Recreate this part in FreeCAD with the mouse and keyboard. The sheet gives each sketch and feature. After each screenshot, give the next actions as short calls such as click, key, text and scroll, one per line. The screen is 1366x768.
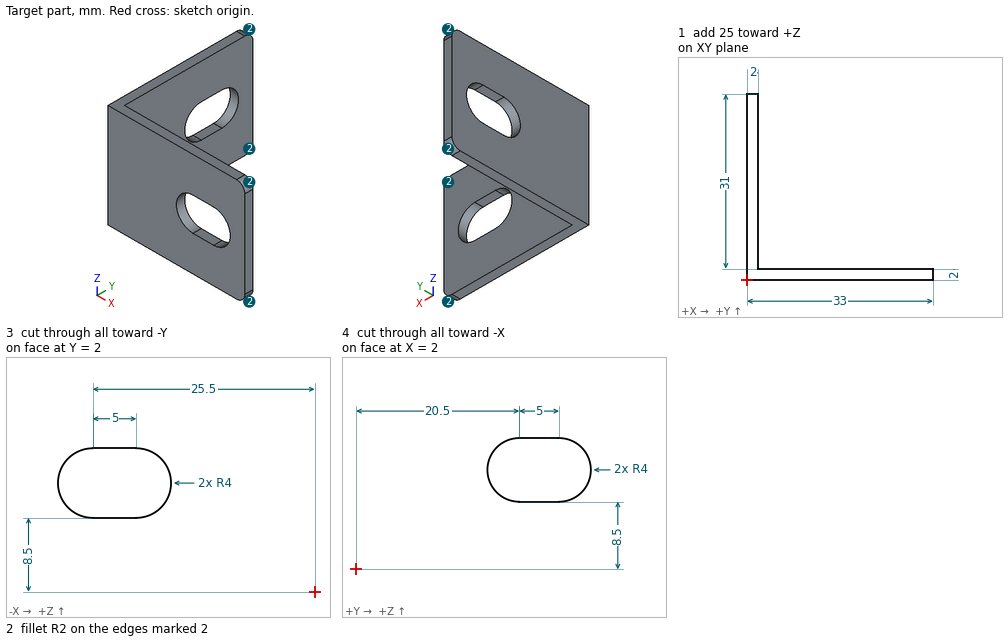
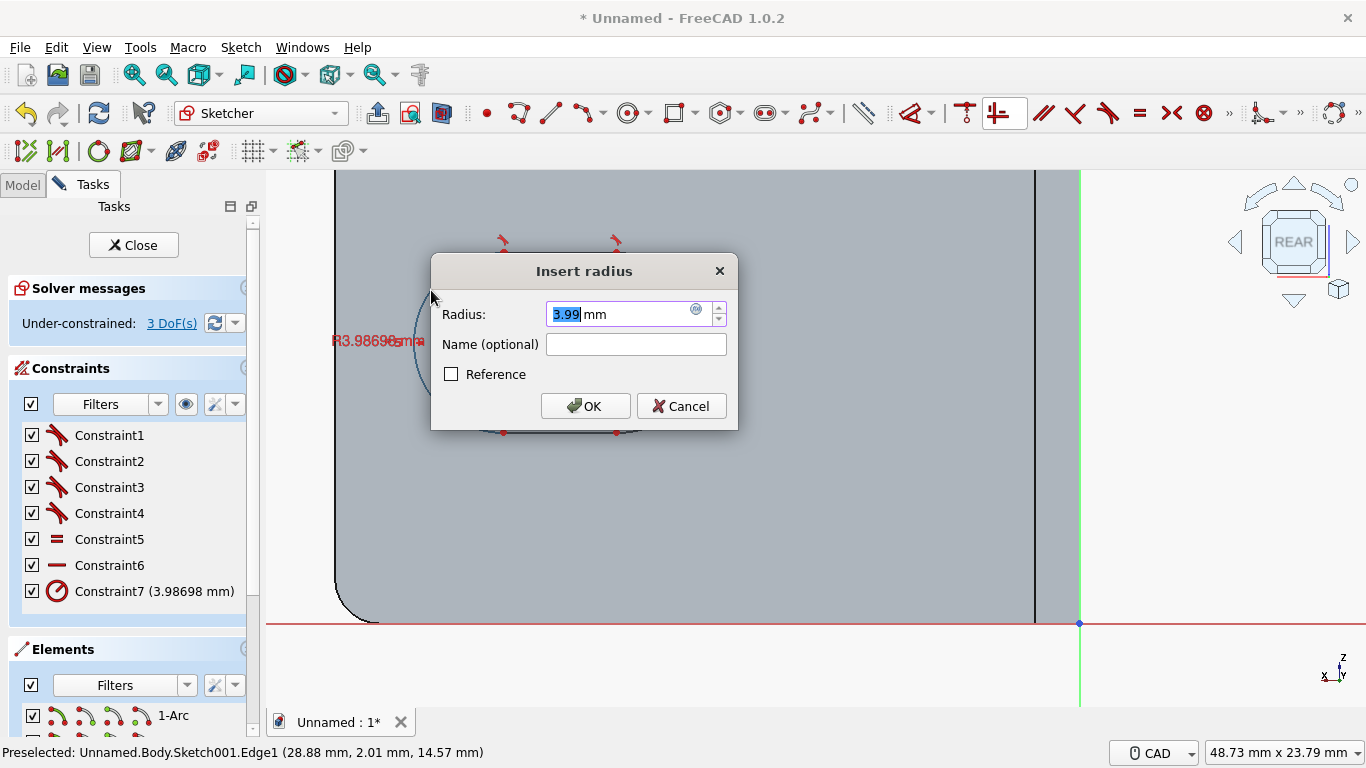
text(4)
key(Return)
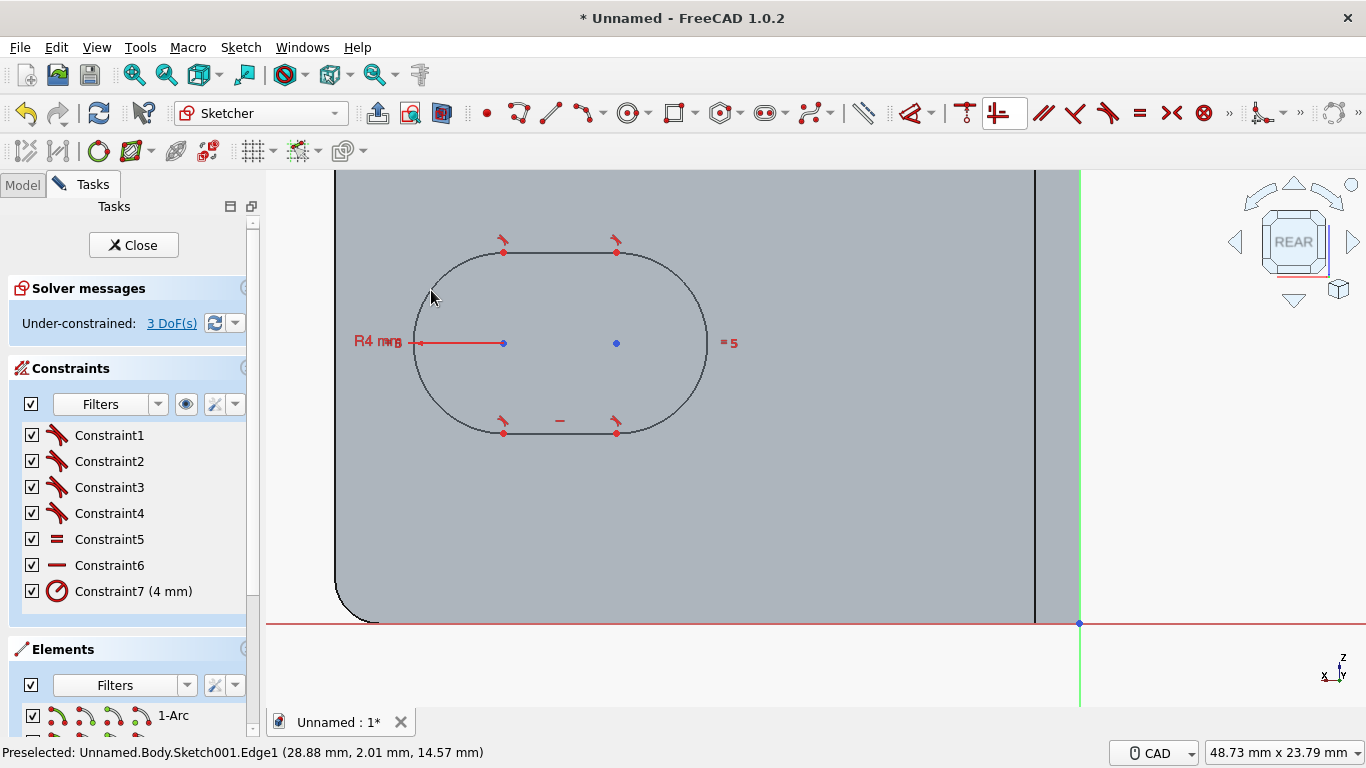
click(538, 253)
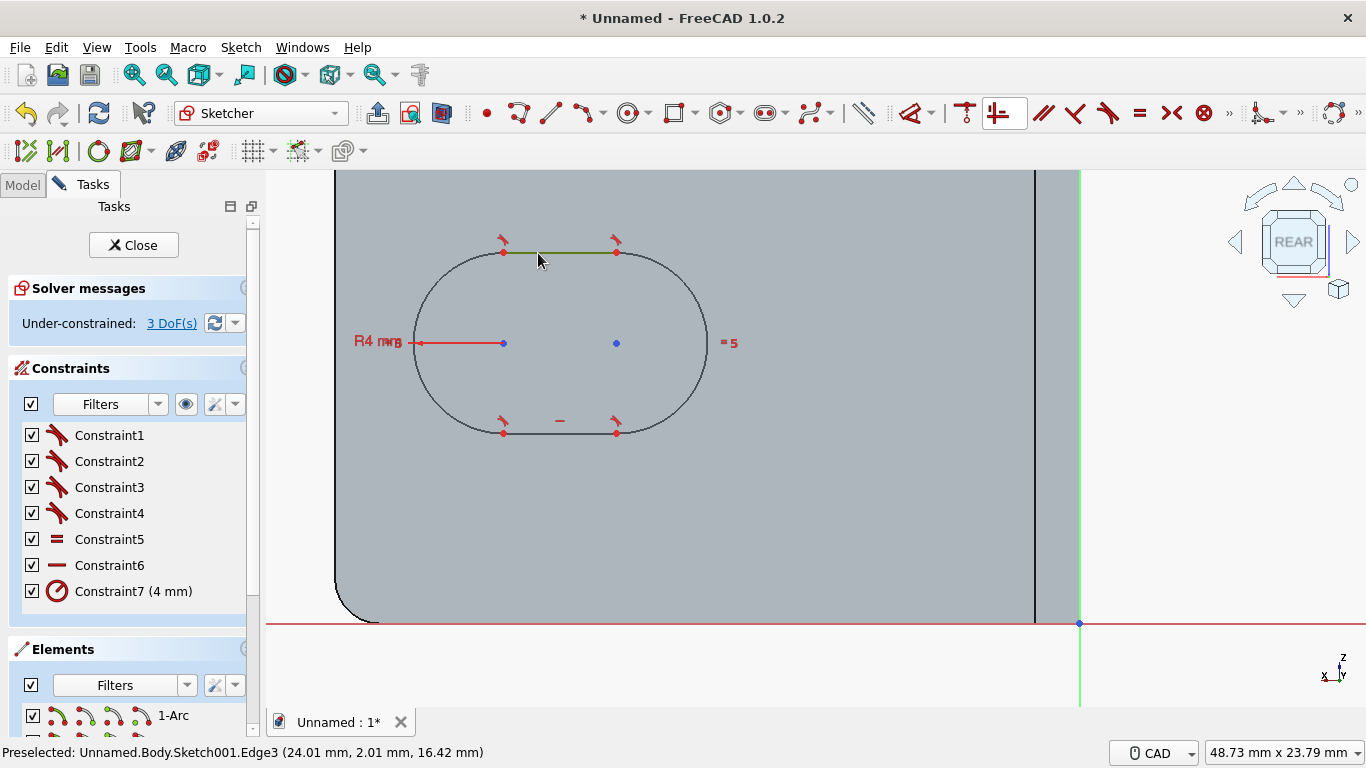
key(l)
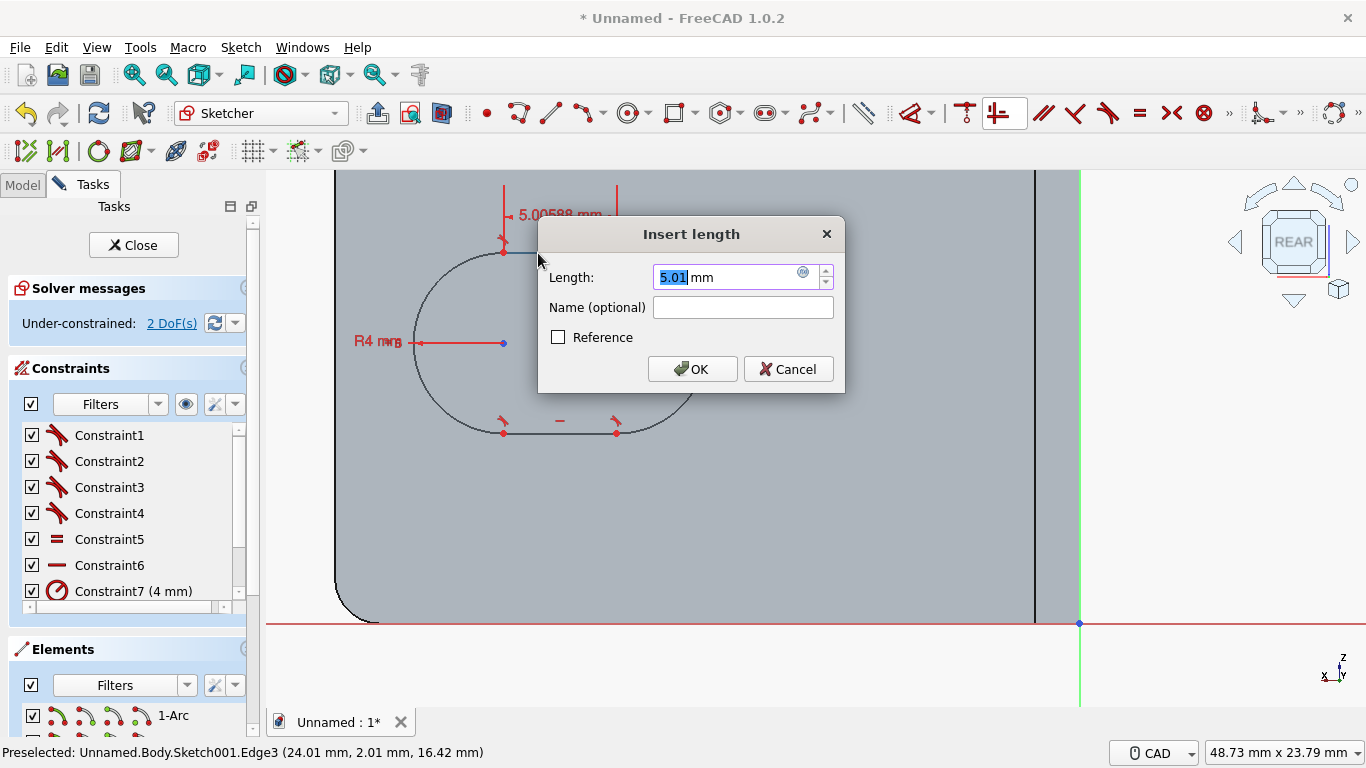
text(5)
key(Return)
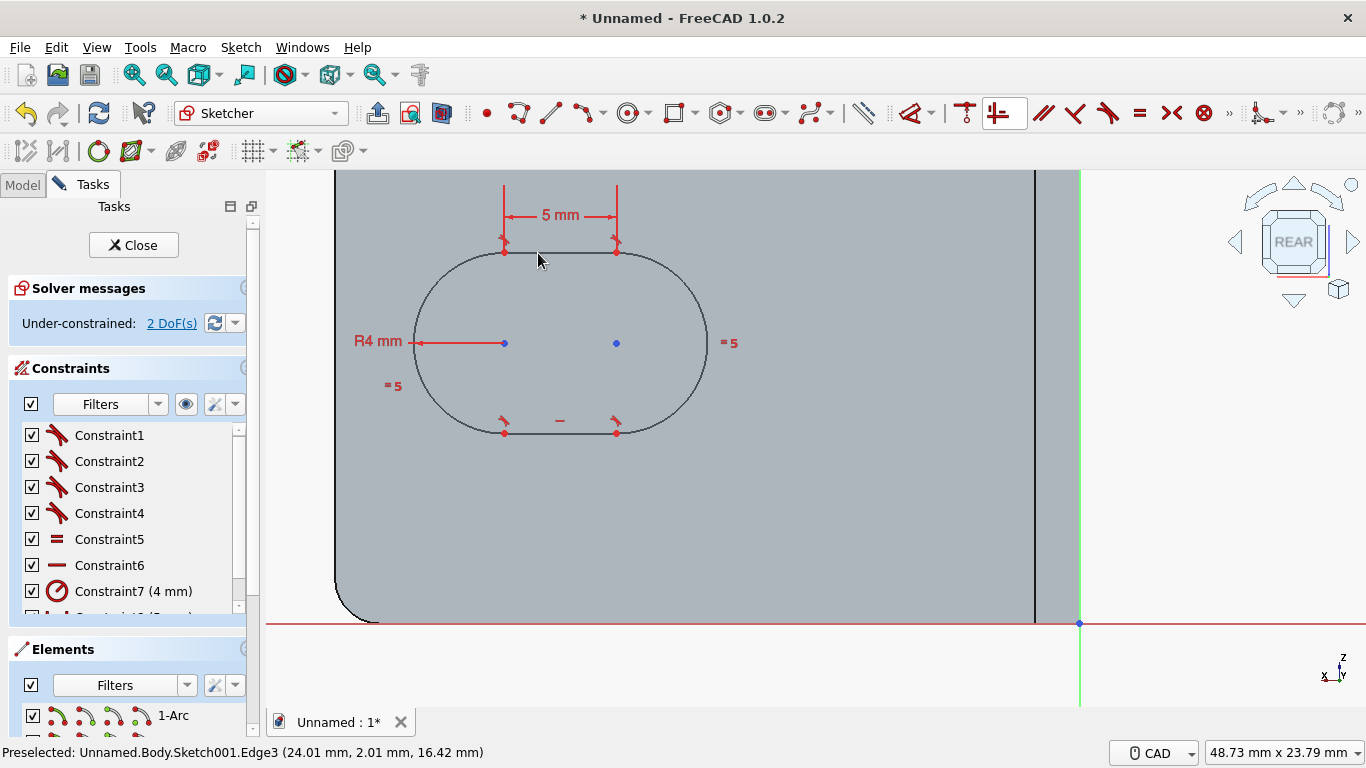
click(504, 434)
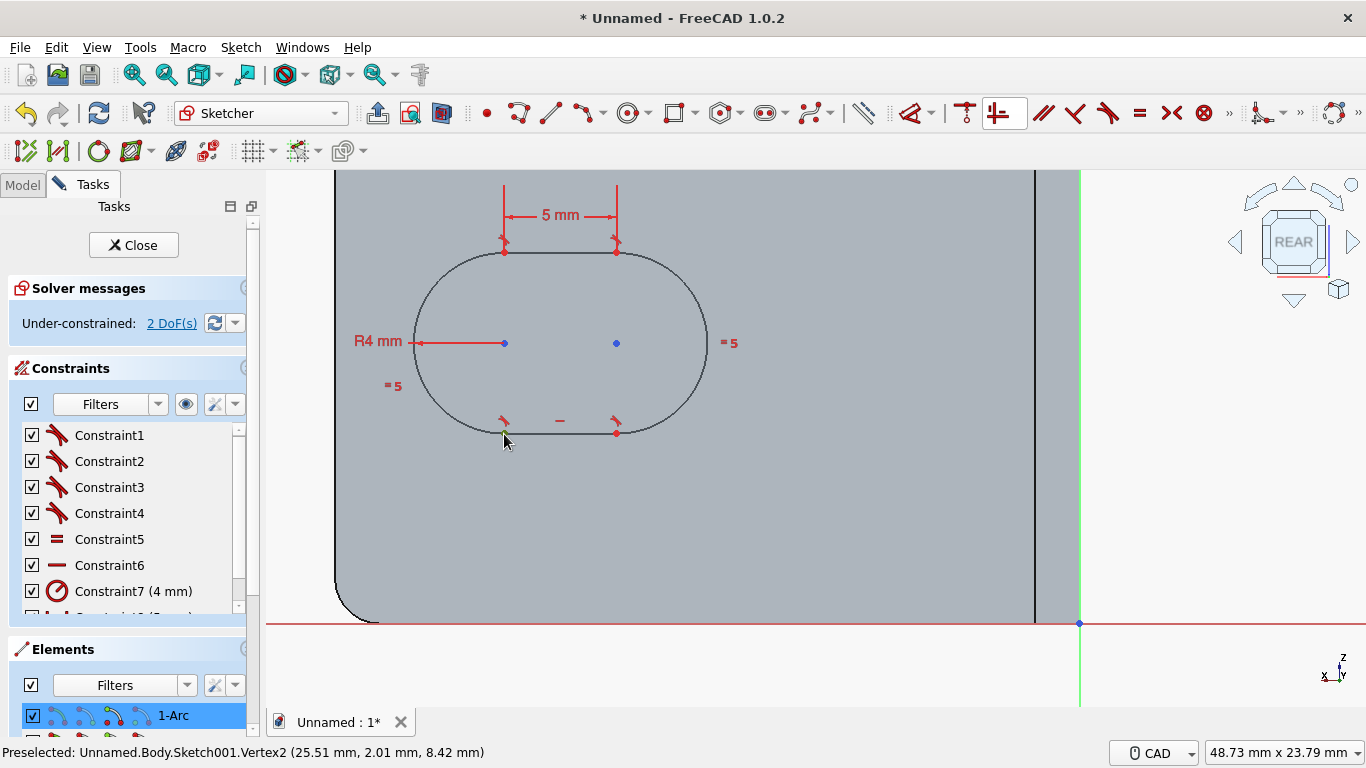
key(i)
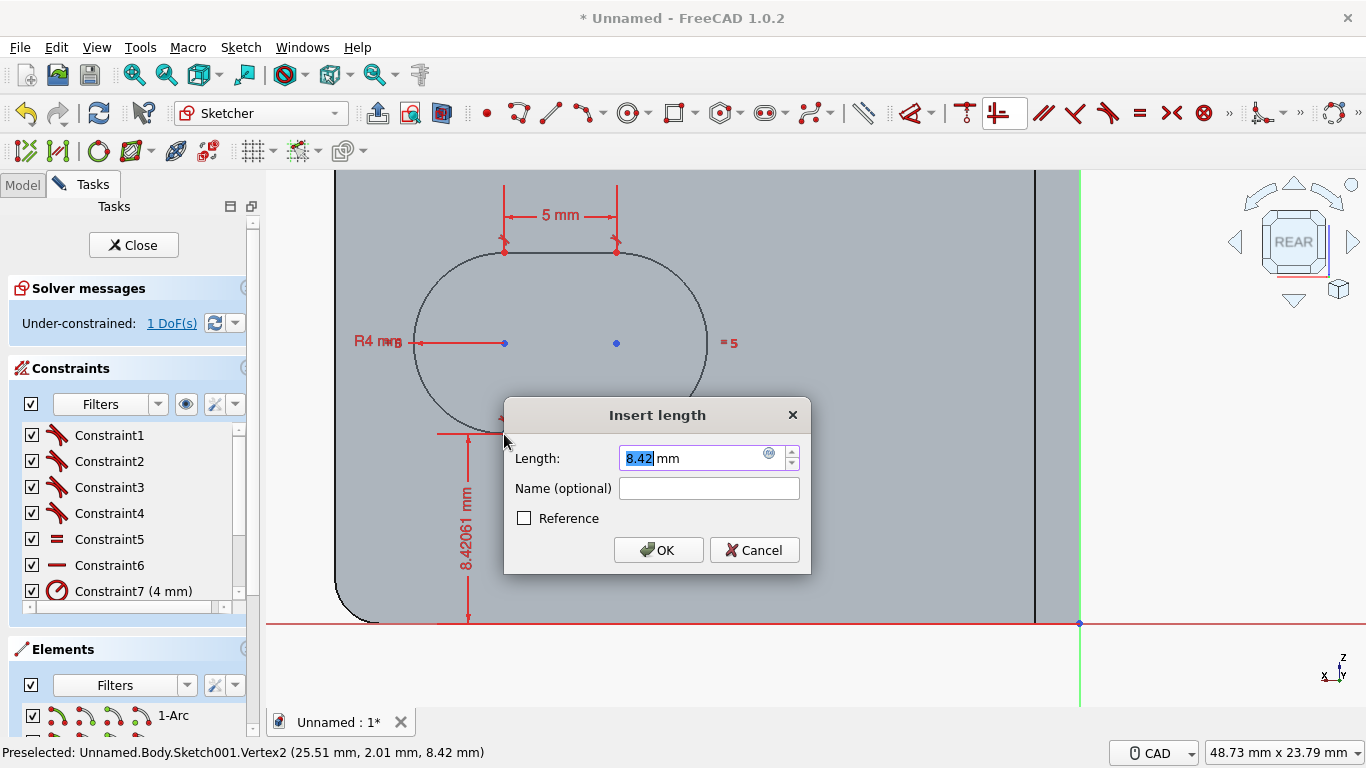
text(8.5)
key(Return)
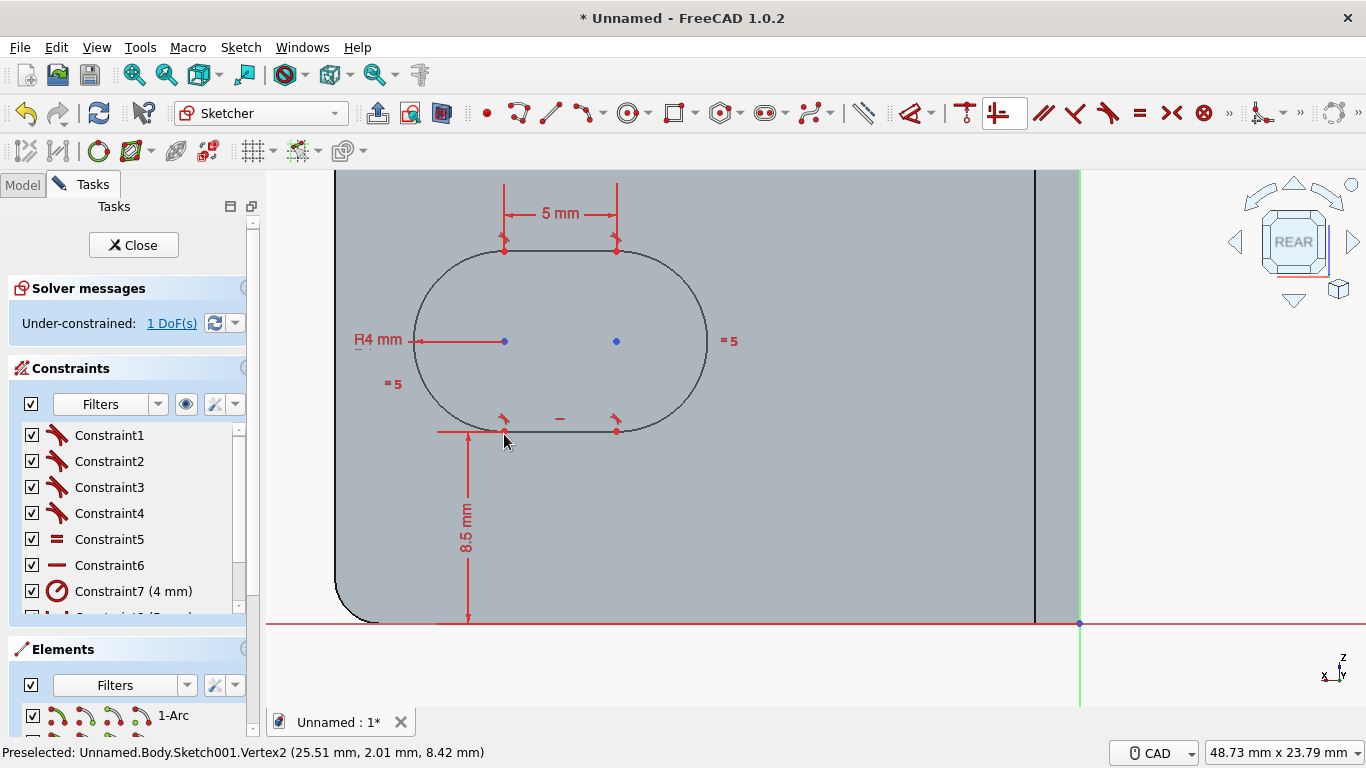
click(504, 251)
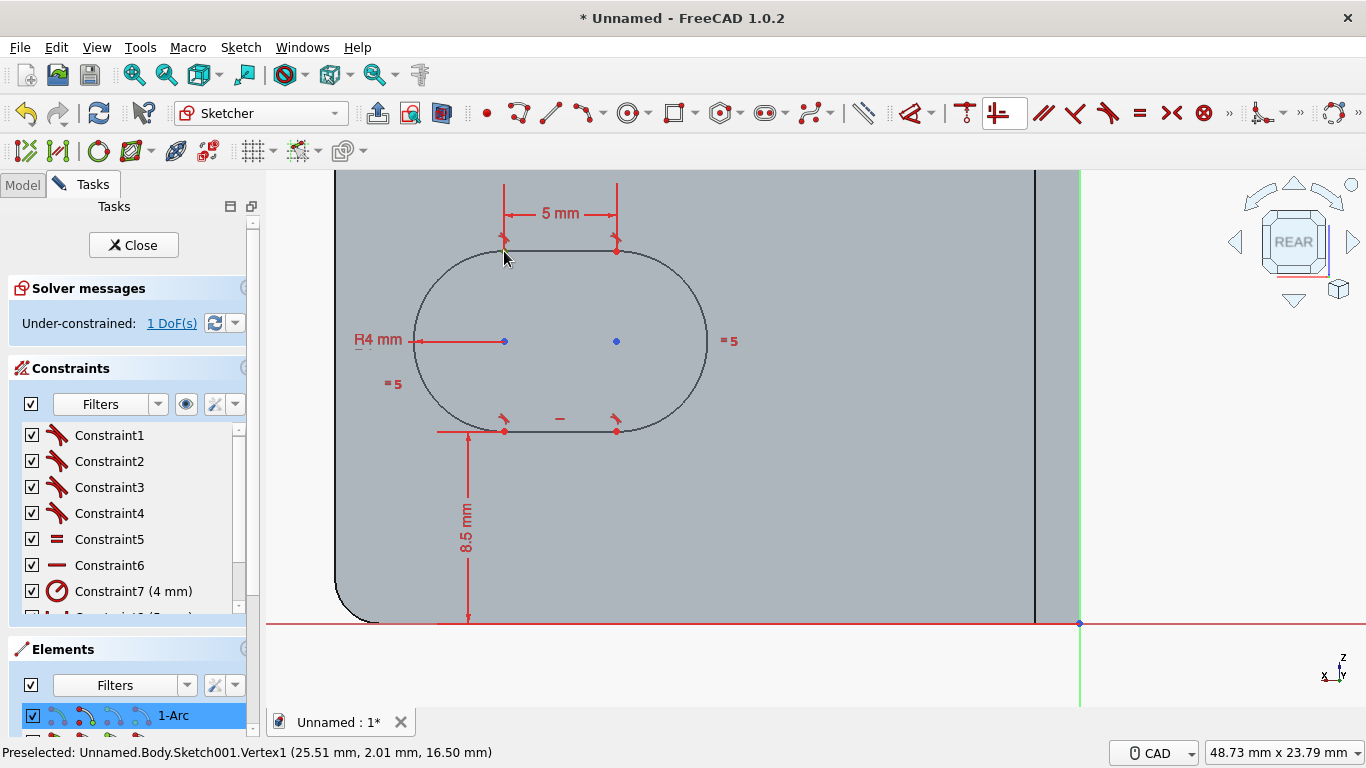
key(l)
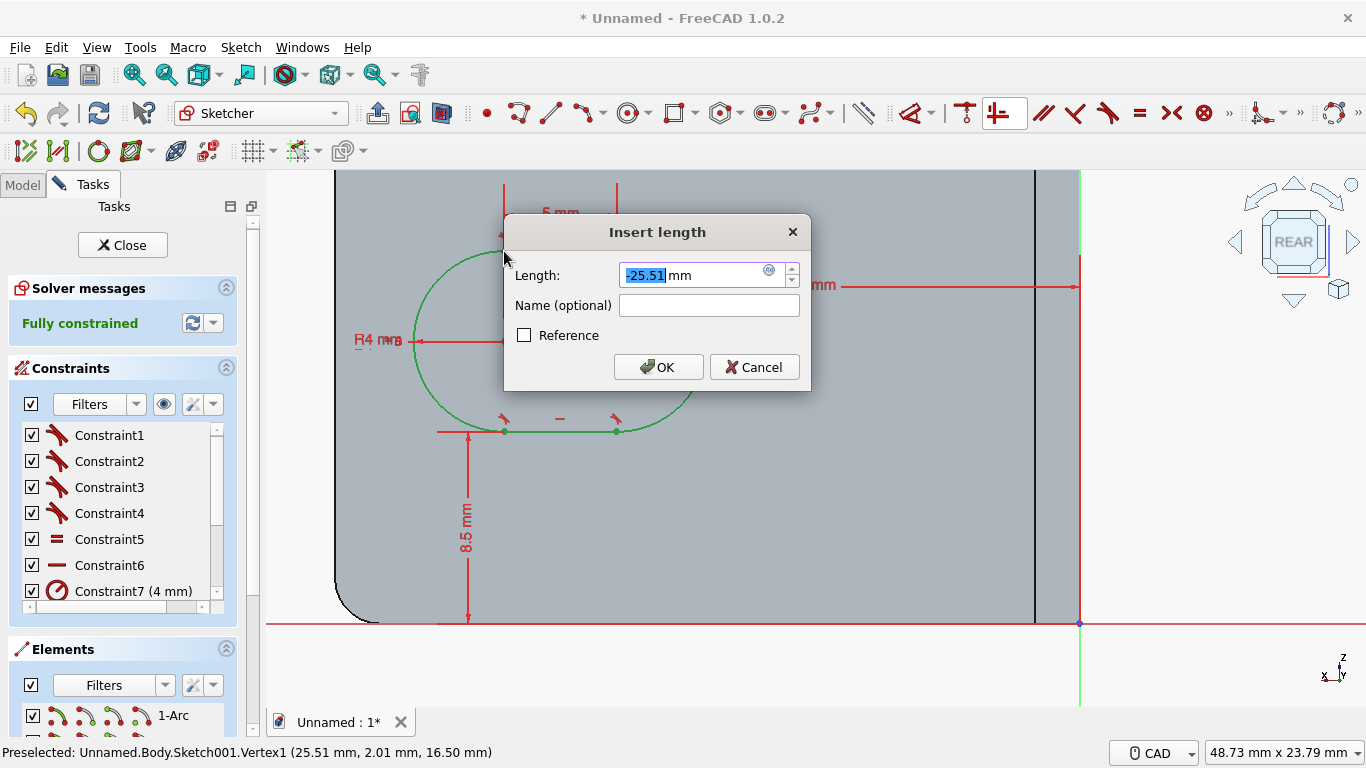
text(-25.5)
key(Return)